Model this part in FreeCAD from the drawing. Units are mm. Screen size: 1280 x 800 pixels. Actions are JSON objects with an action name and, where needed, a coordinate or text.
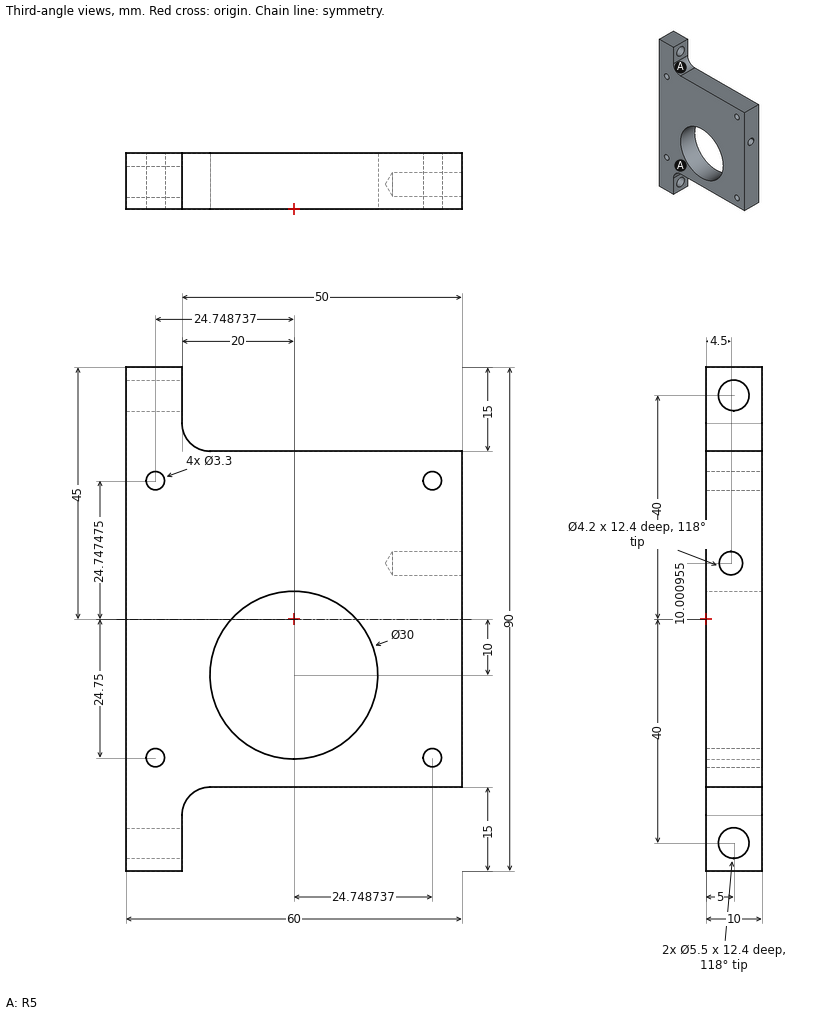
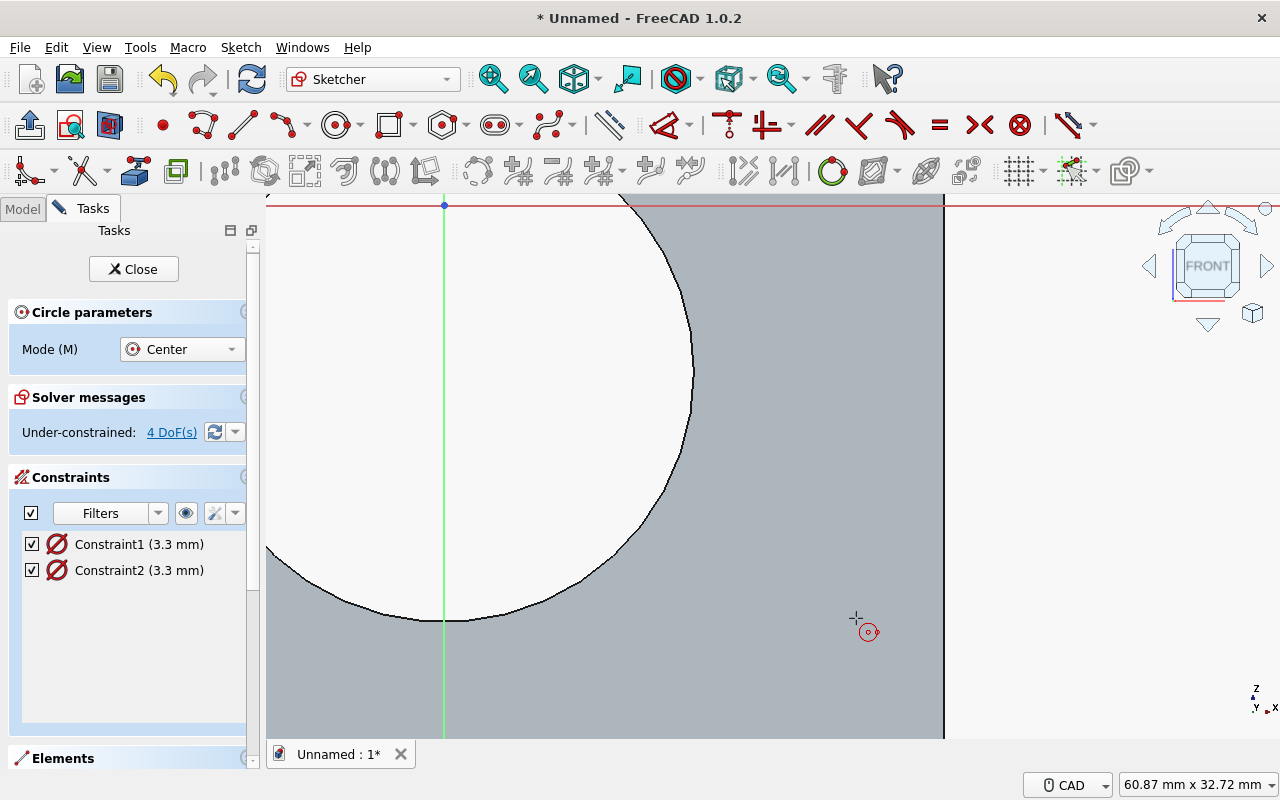
{"action": "left_click", "coordinate": [856, 618]}
{"action": "mouse_move", "coordinate": [876, 598]}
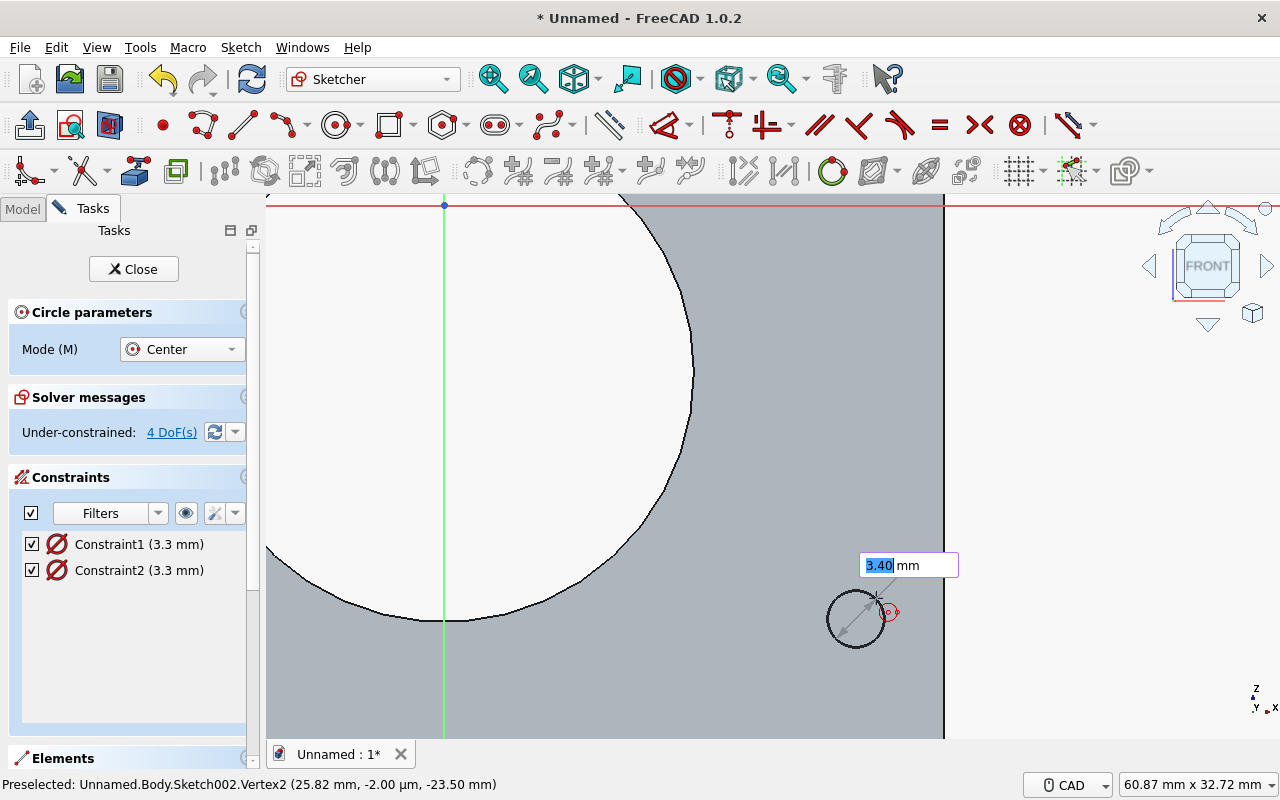
{"action": "type", "text": "3.3"}
{"action": "key", "text": "Return"}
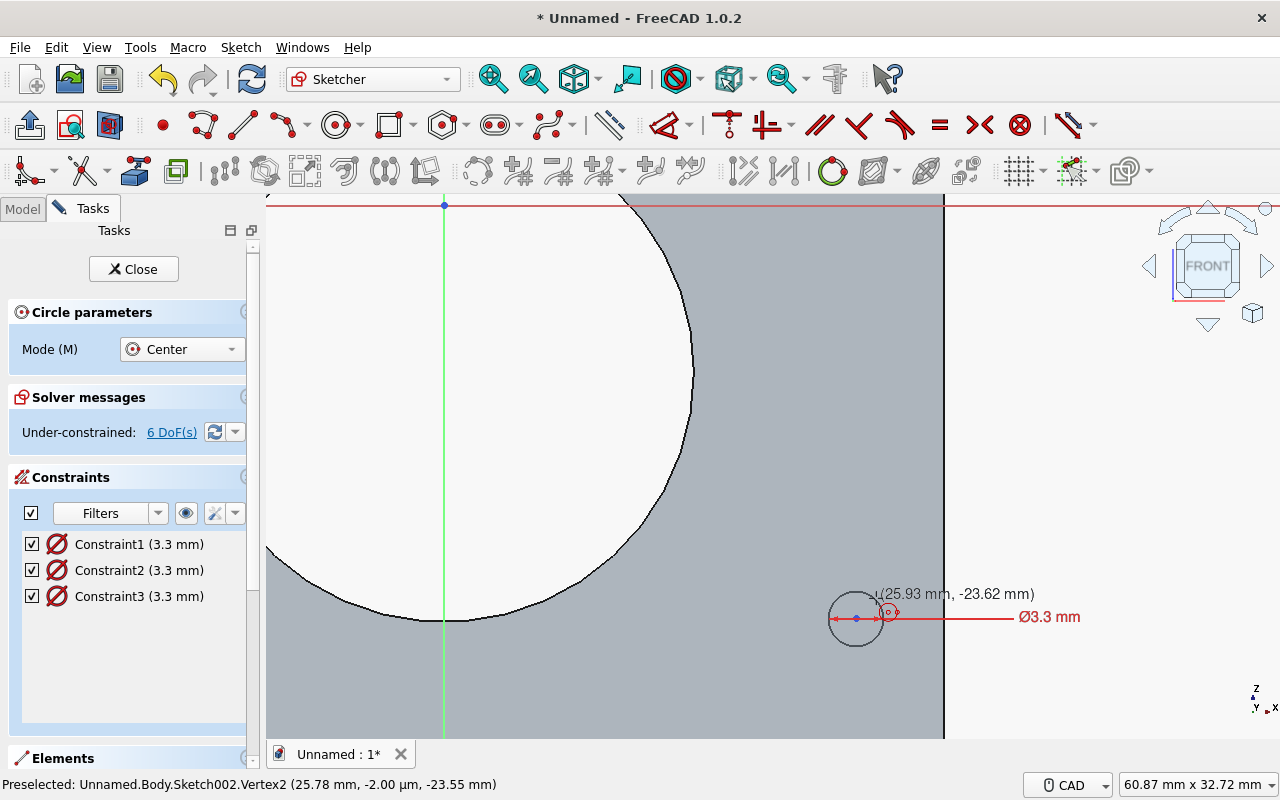
{"action": "scroll", "coordinate": [856, 618], "scroll_direction": "down", "scroll_amount": 5}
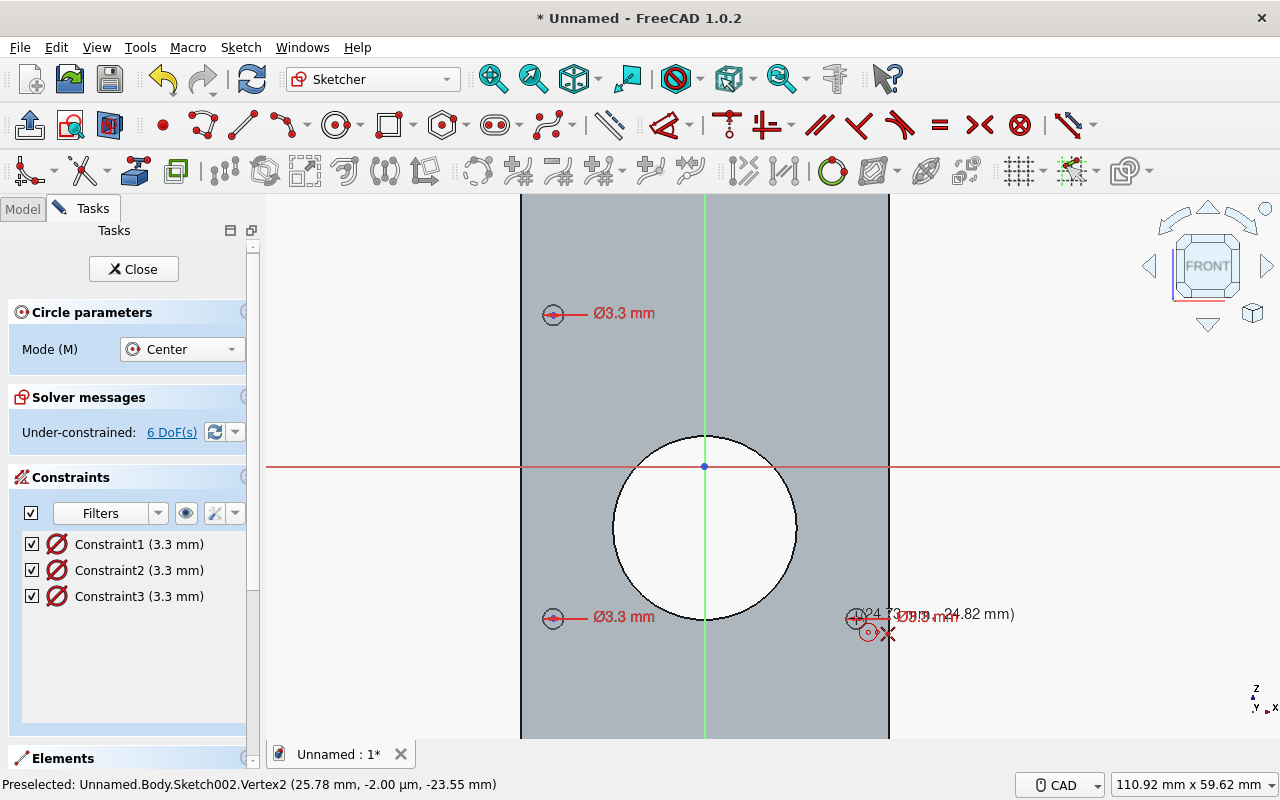
{"action": "scroll", "coordinate": [856, 315], "scroll_direction": "up", "scroll_amount": 5}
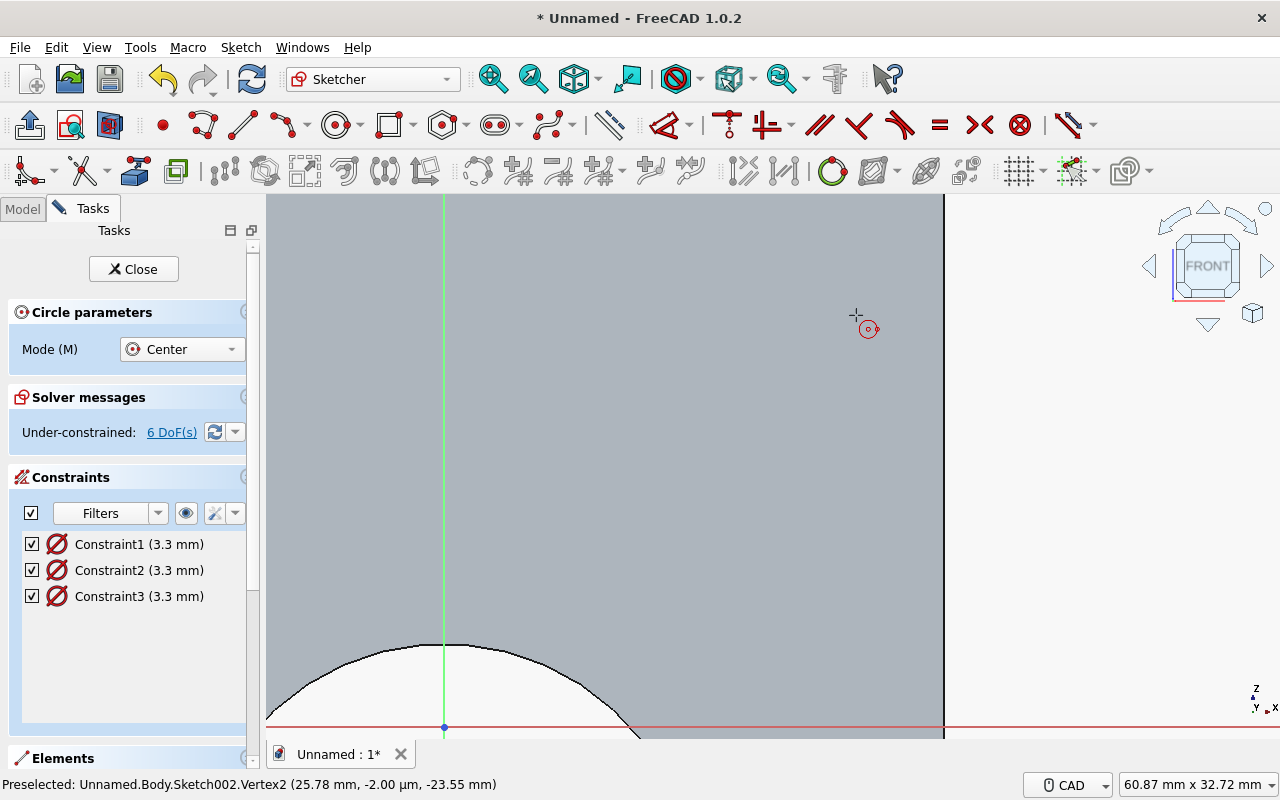
{"action": "left_click", "coordinate": [856, 315]}
{"action": "mouse_move", "coordinate": [876, 296]}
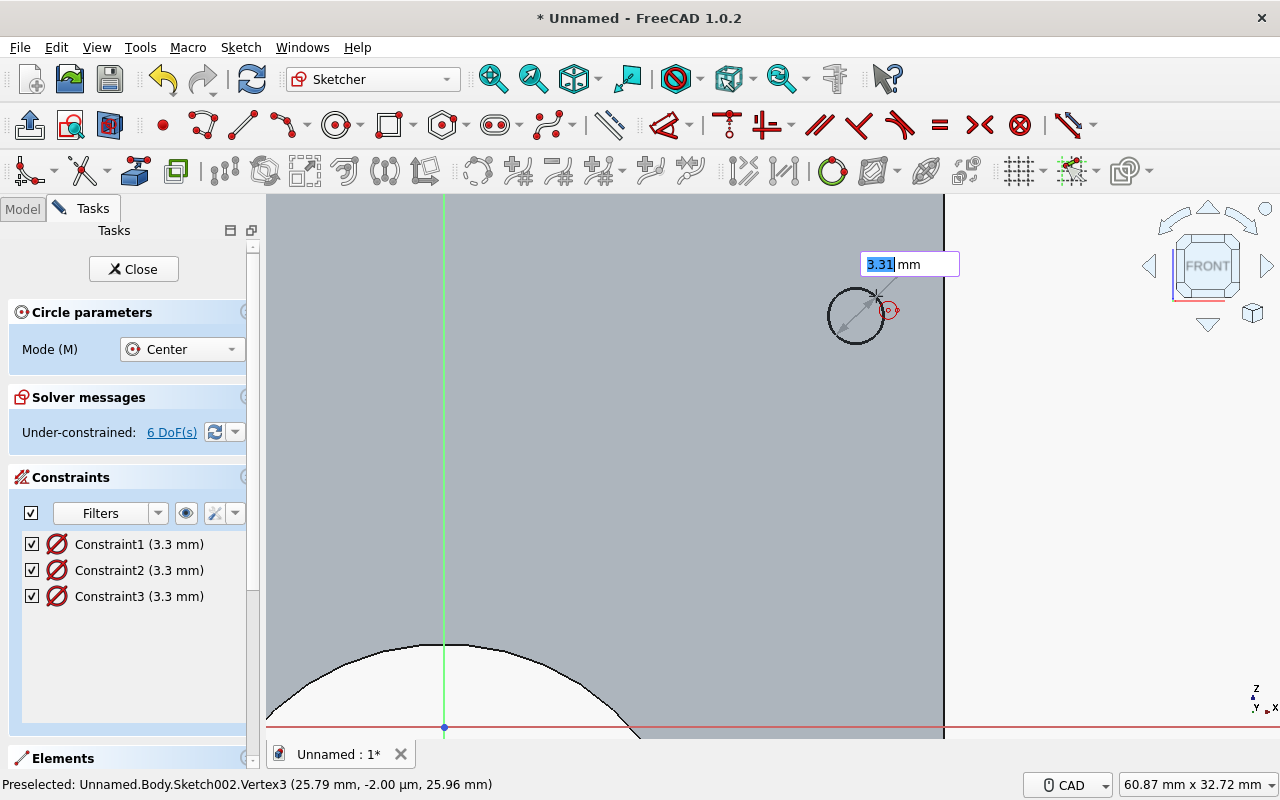
{"action": "type", "text": "3.3"}
{"action": "key", "text": "Return"}
{"action": "key", "text": "Escape"}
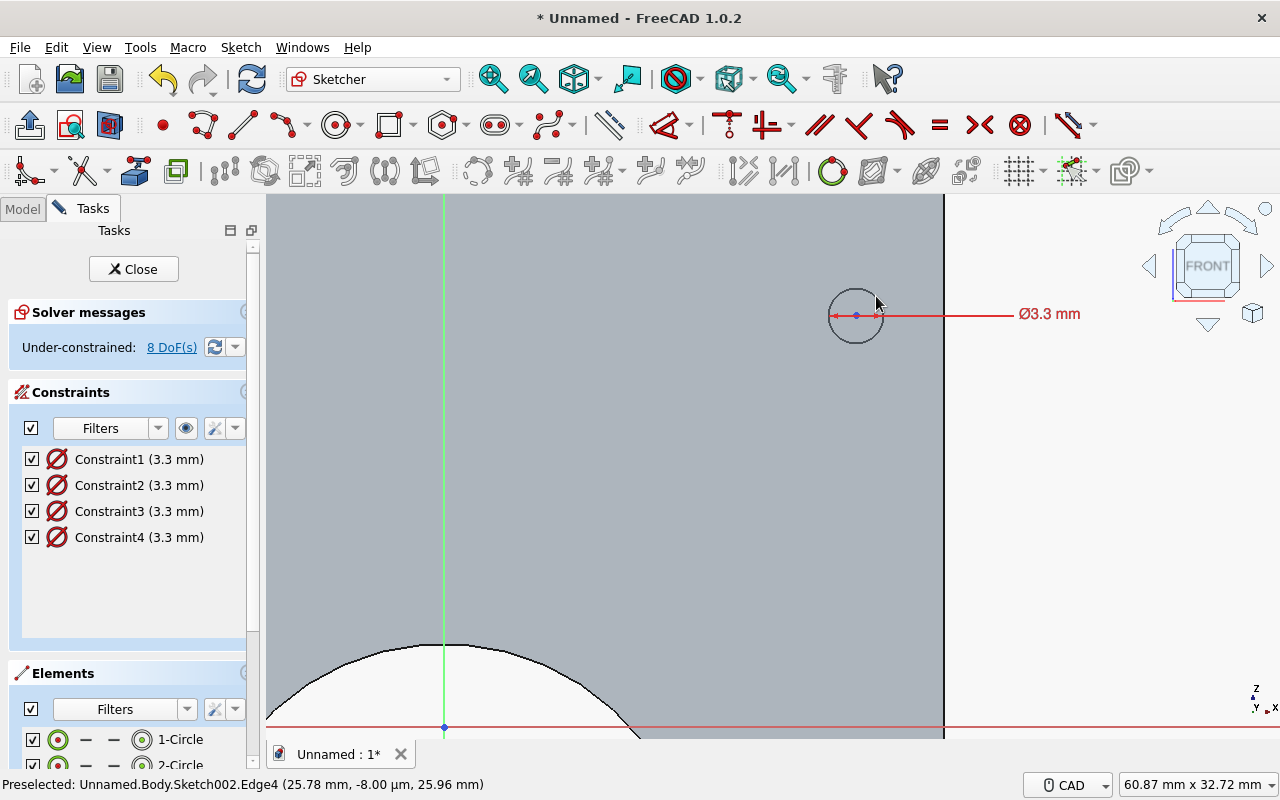
{"action": "scroll", "coordinate": [856, 315], "scroll_direction": "down", "scroll_amount": 5}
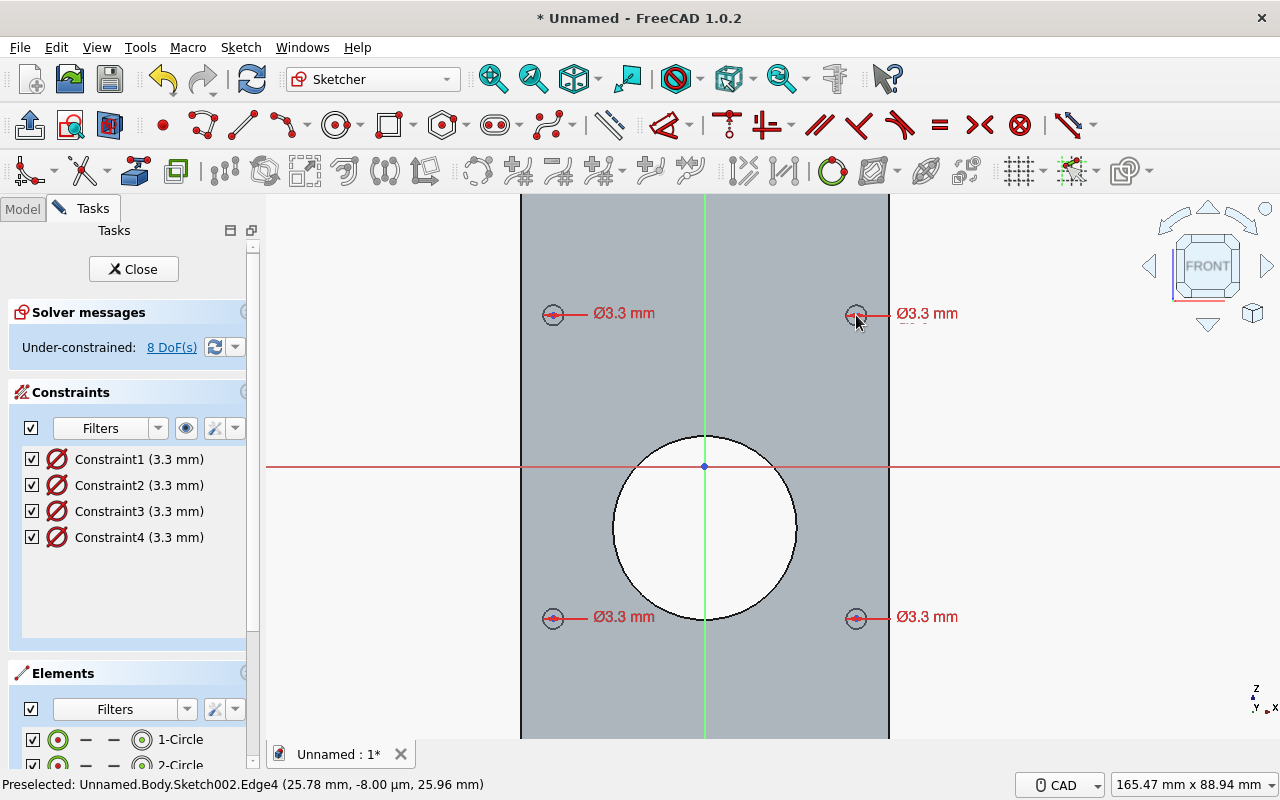
{"action": "left_click", "coordinate": [553, 315]}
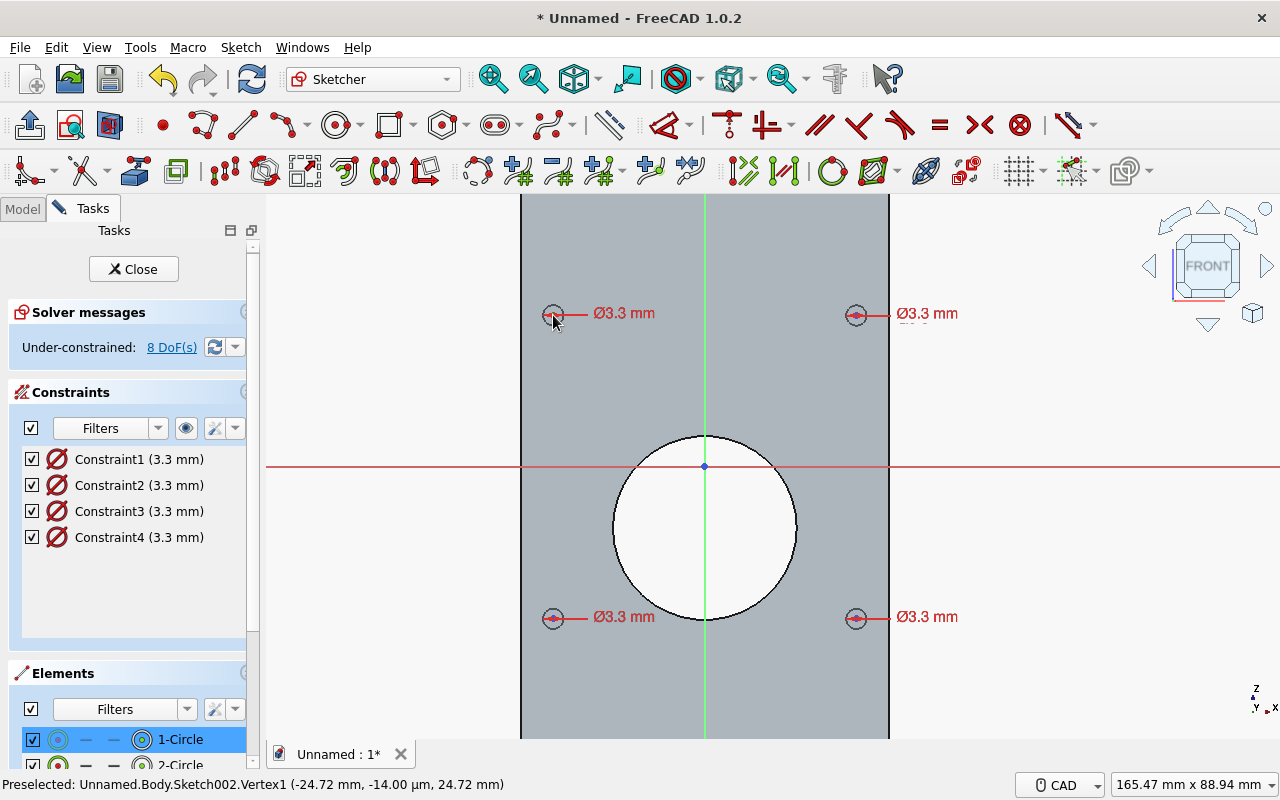
{"action": "left_click", "coordinate": [553, 619]}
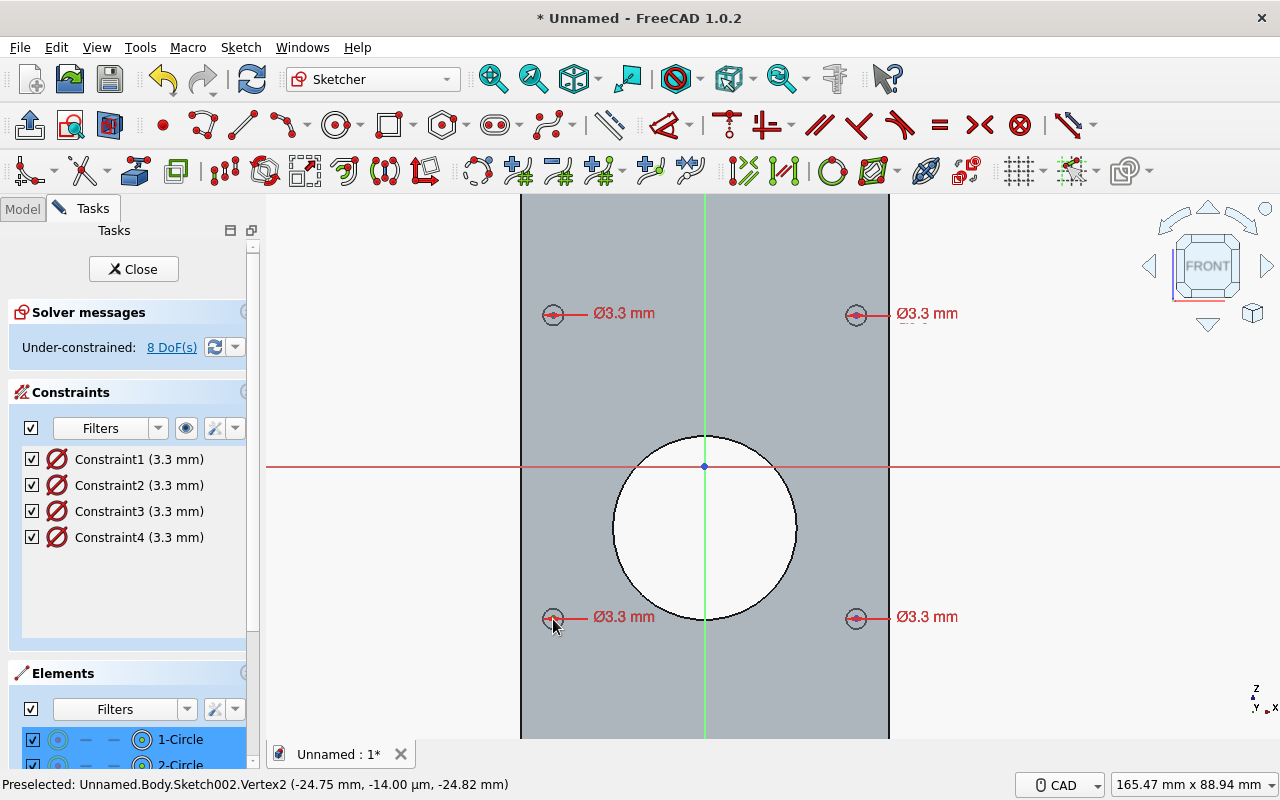
{"action": "key", "text": "v"}